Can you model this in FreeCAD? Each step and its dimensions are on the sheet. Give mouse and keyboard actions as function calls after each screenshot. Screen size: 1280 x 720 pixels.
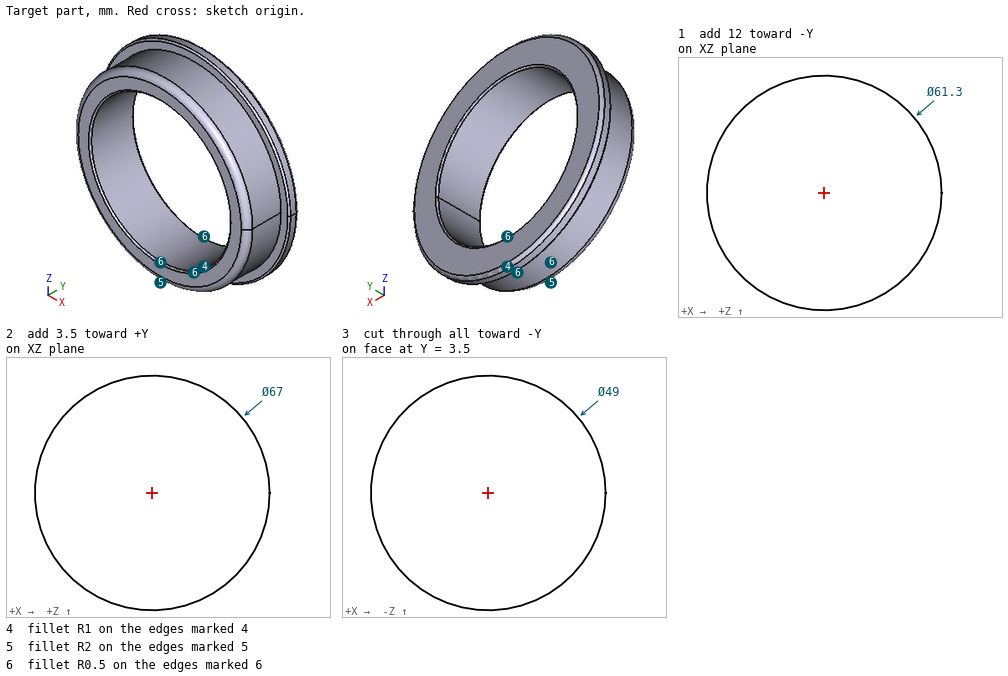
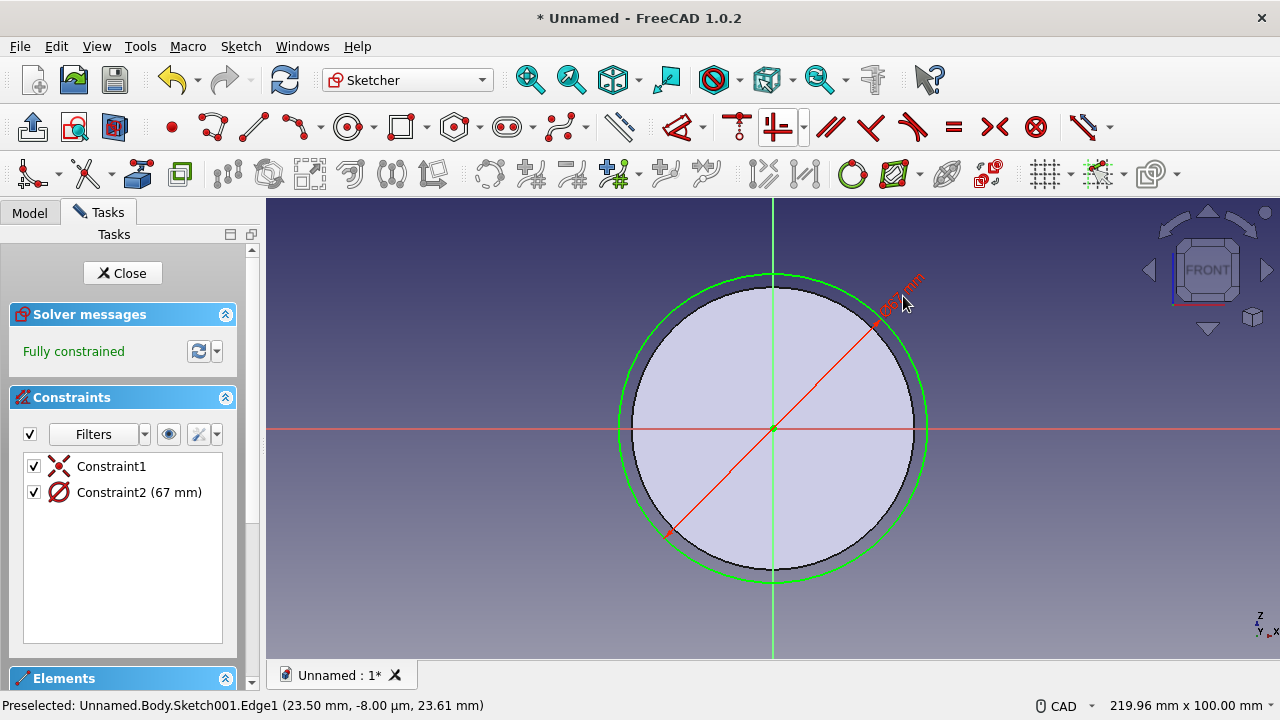
click(123, 273)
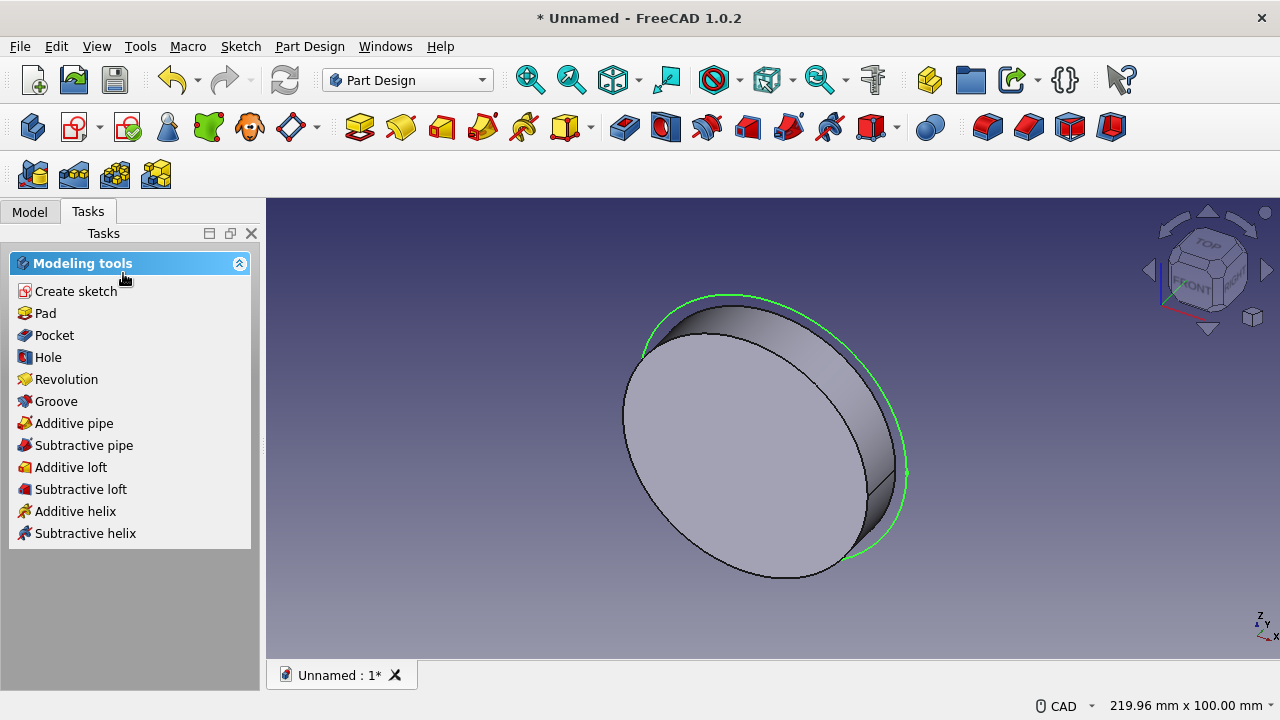
click(360, 128)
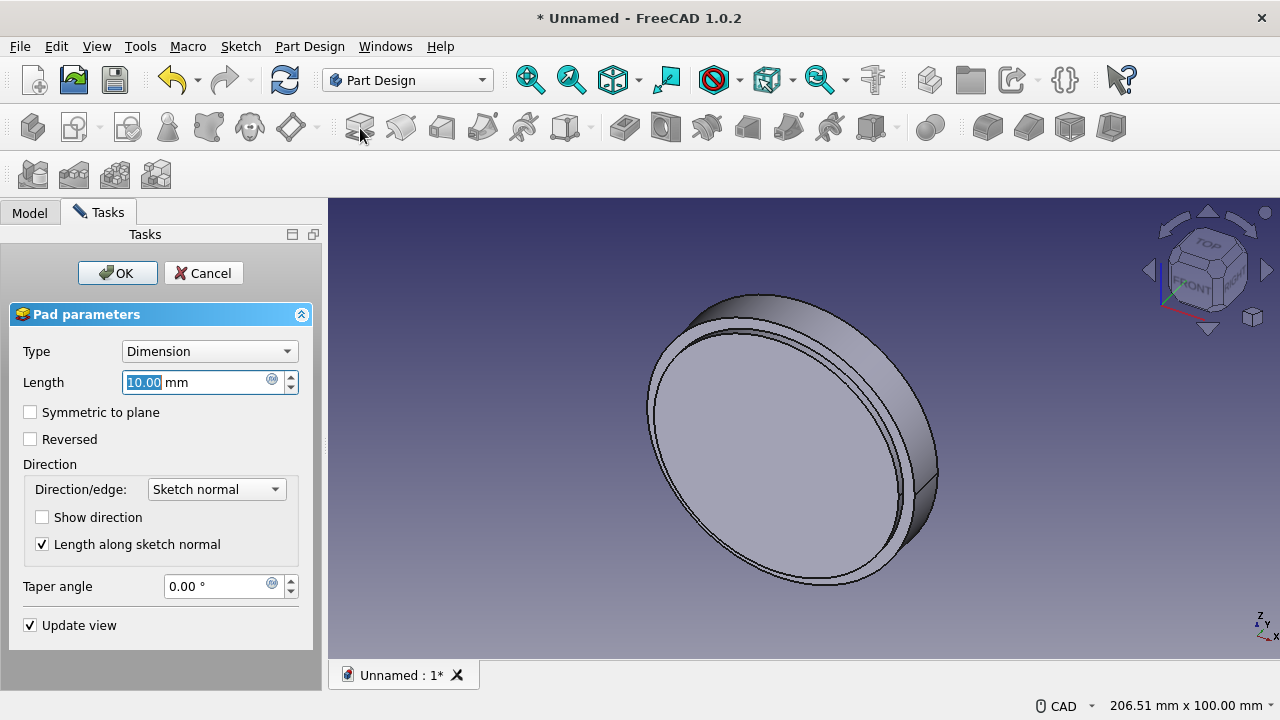
text(3.5)
key(Tab)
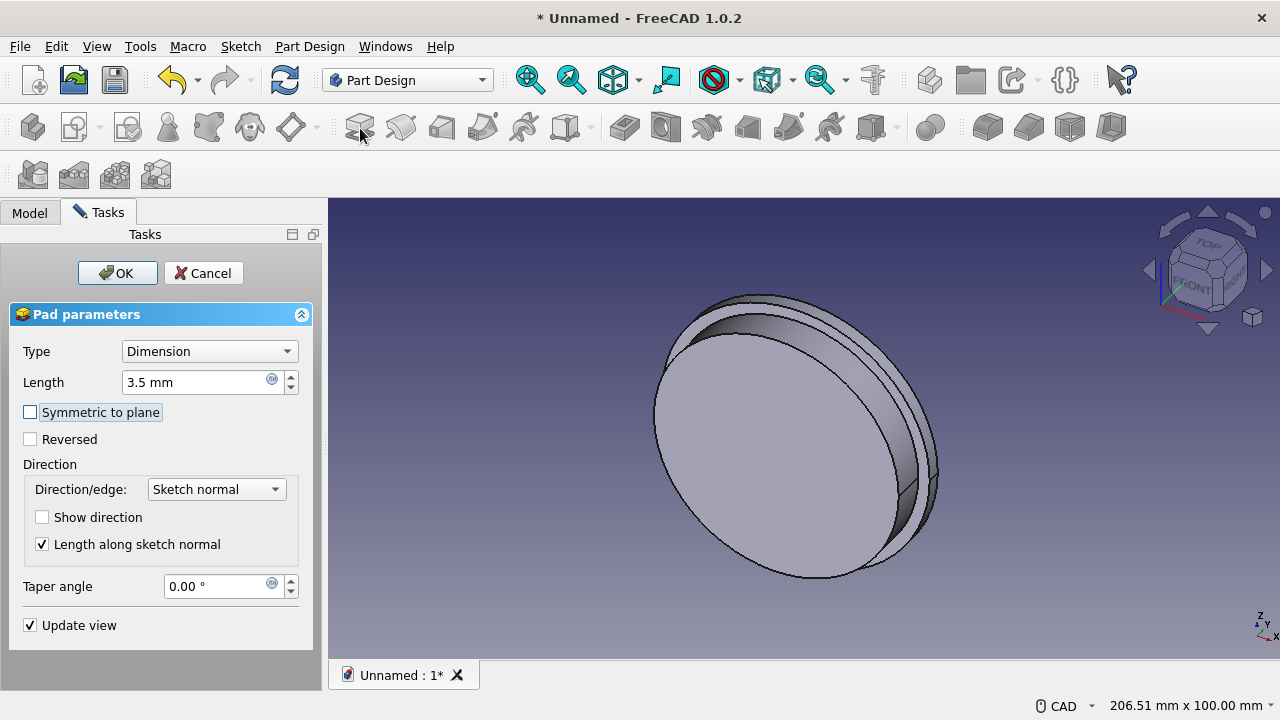
click(31, 439)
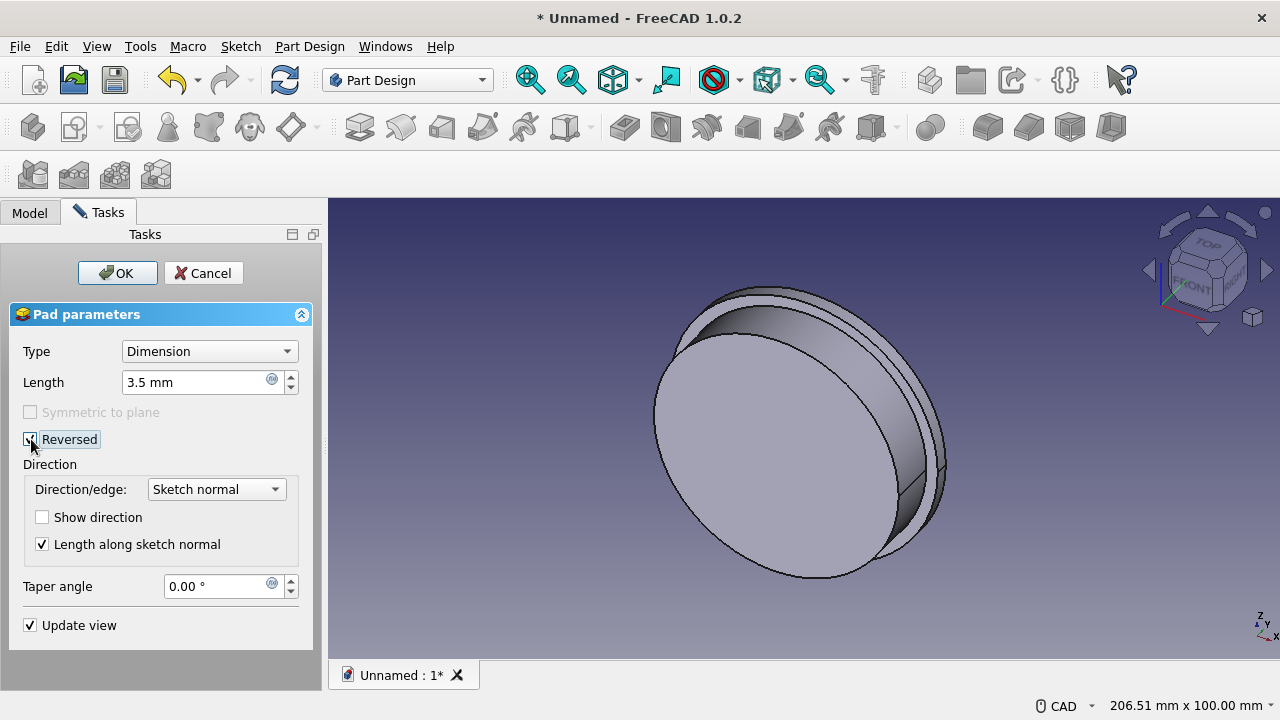
click(118, 273)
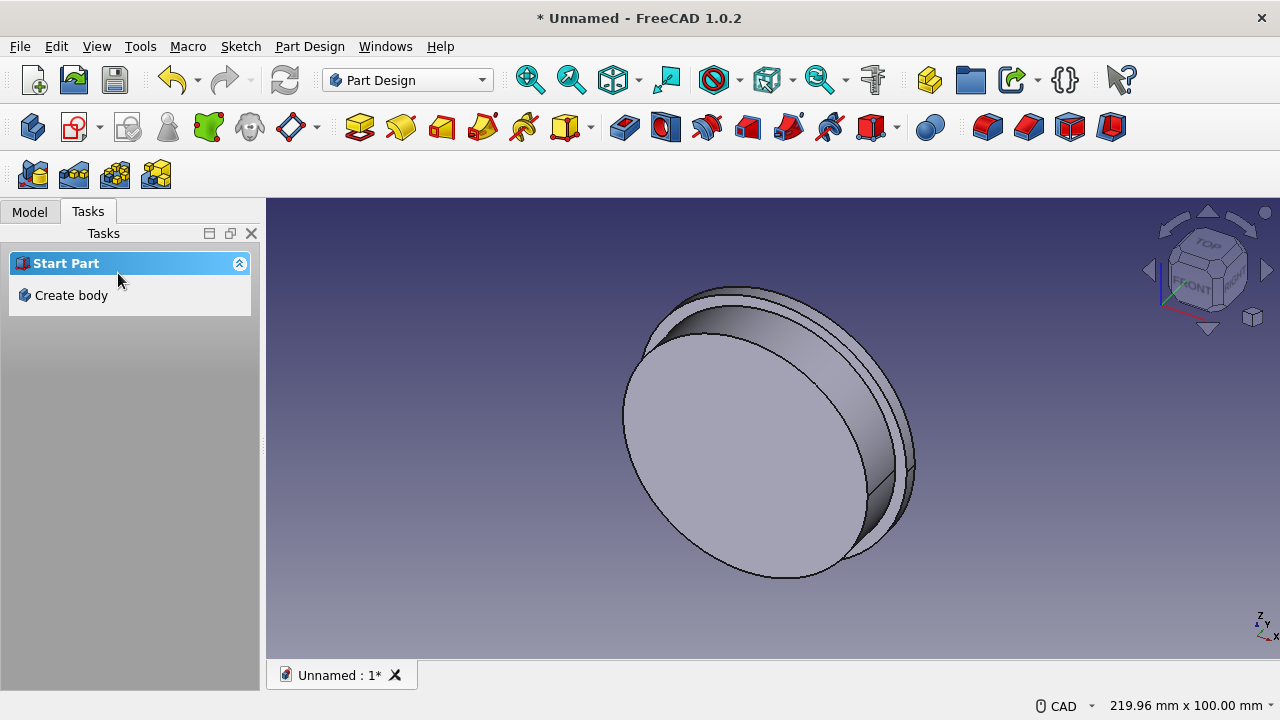
key(4)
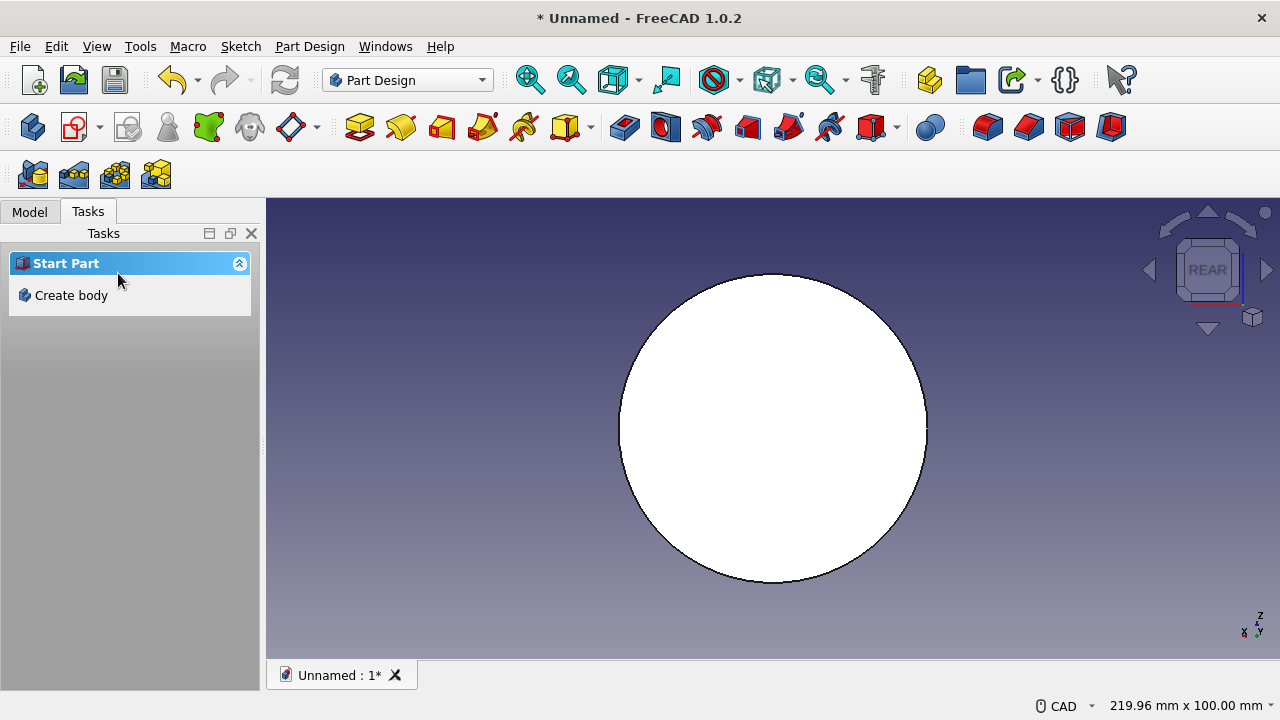
click(773, 427)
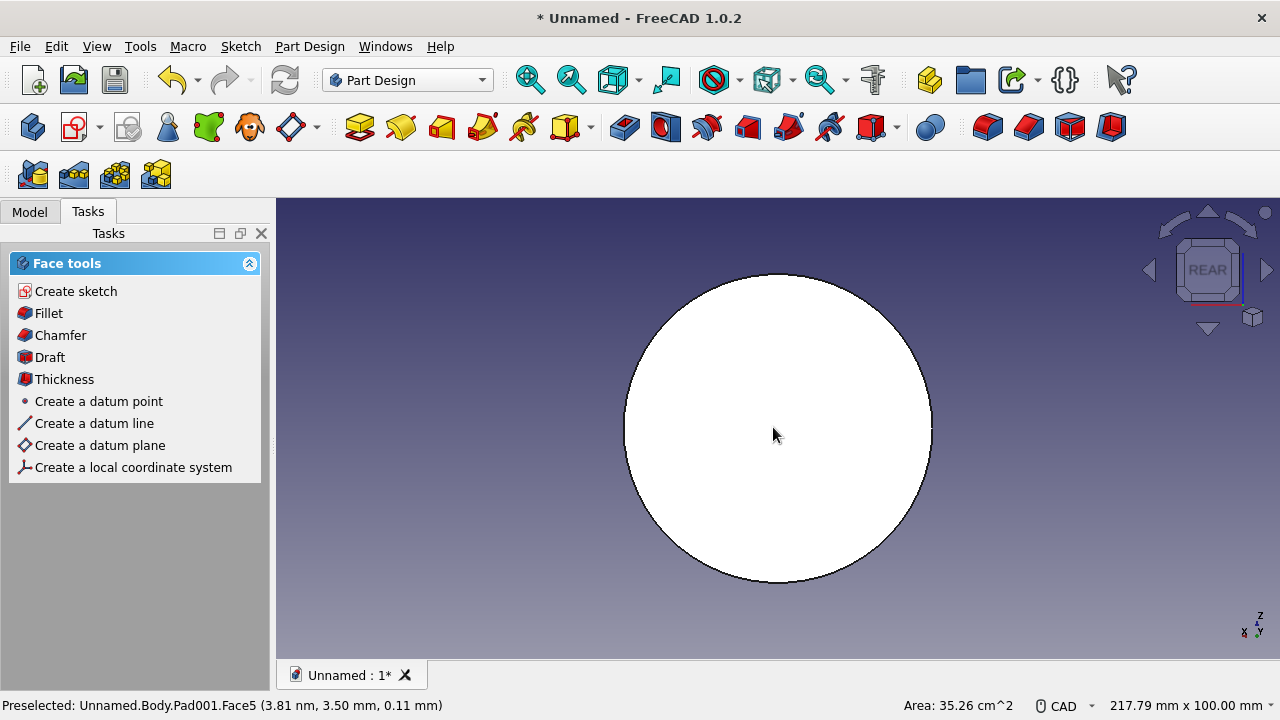
click(74, 128)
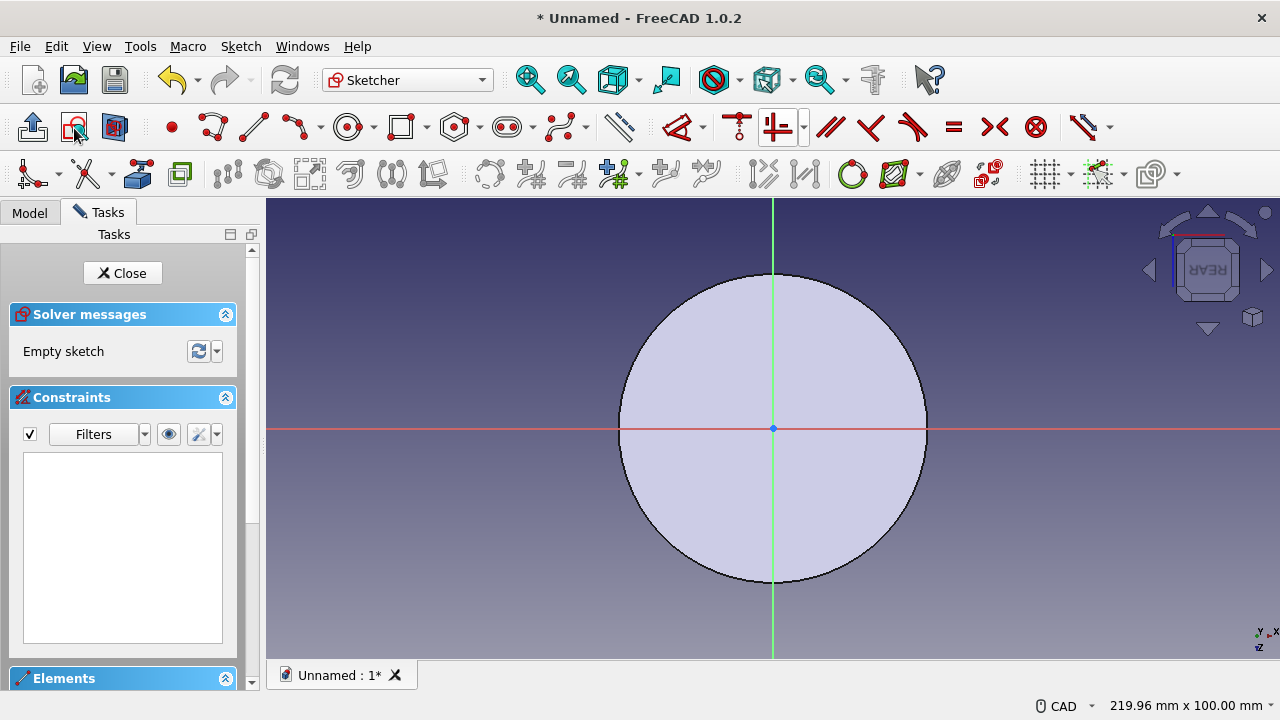
click(348, 128)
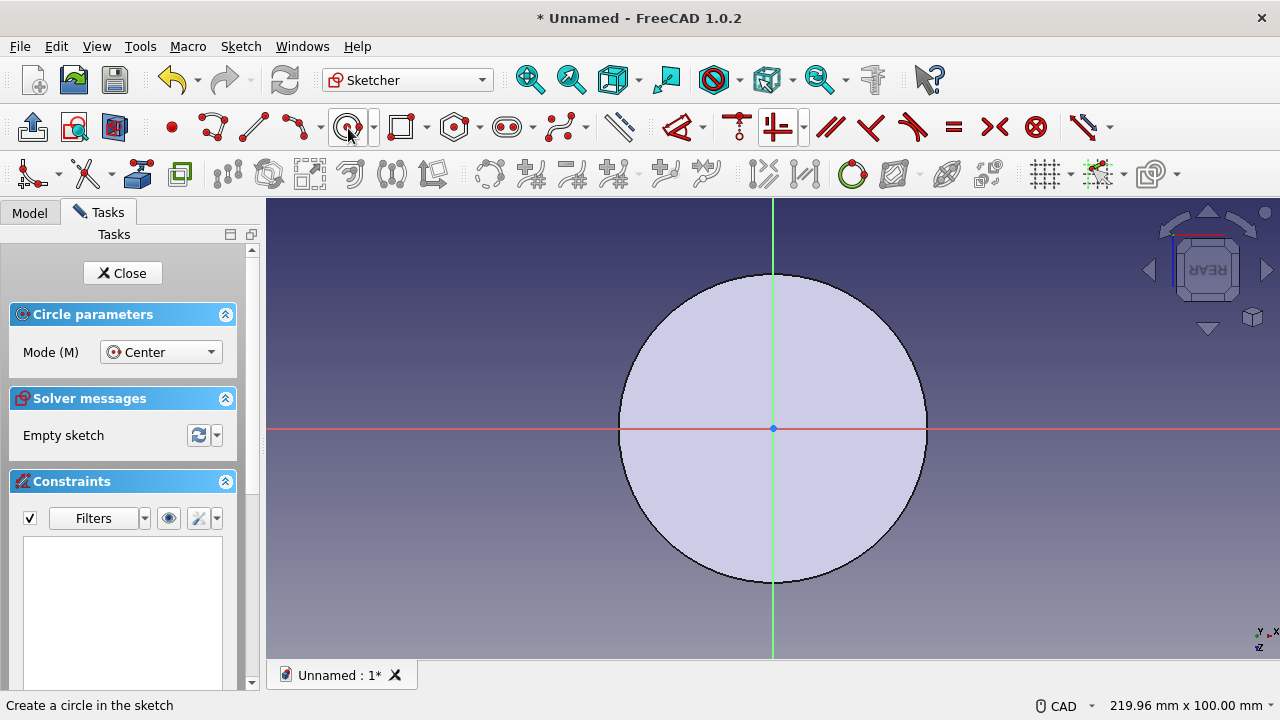
click(773, 429)
click(853, 349)
key(Escape)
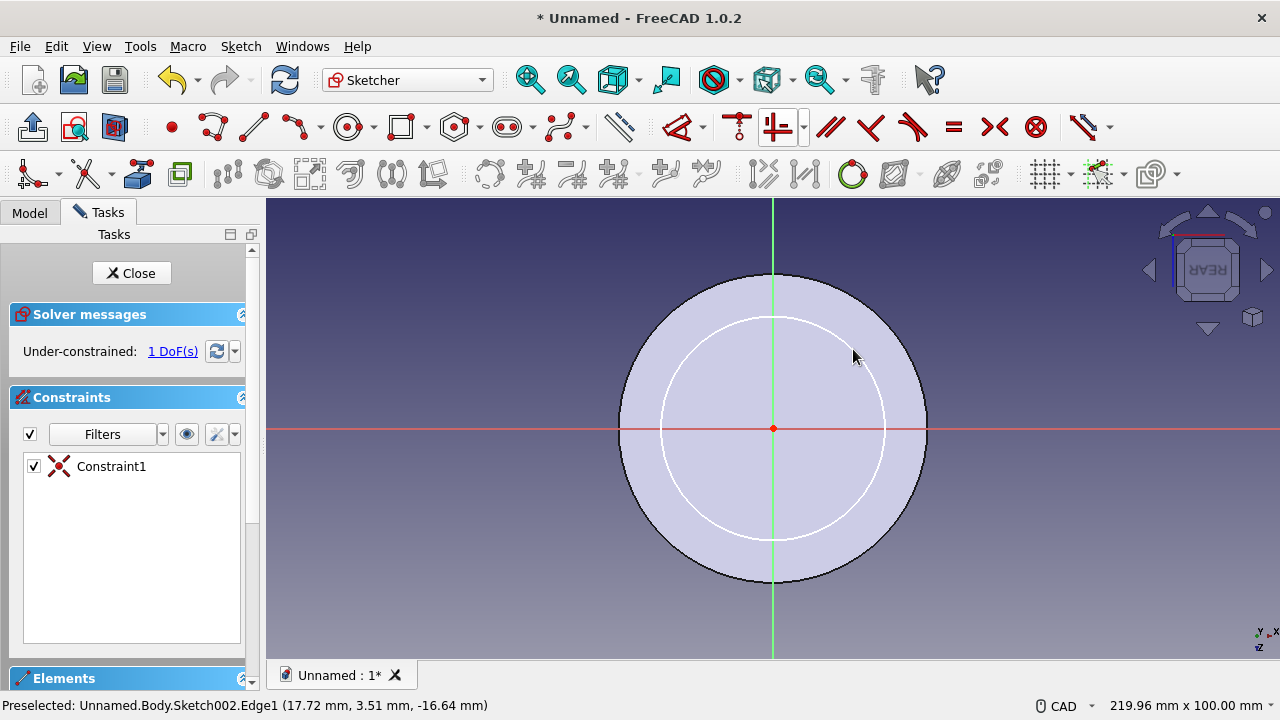
click(676, 128)